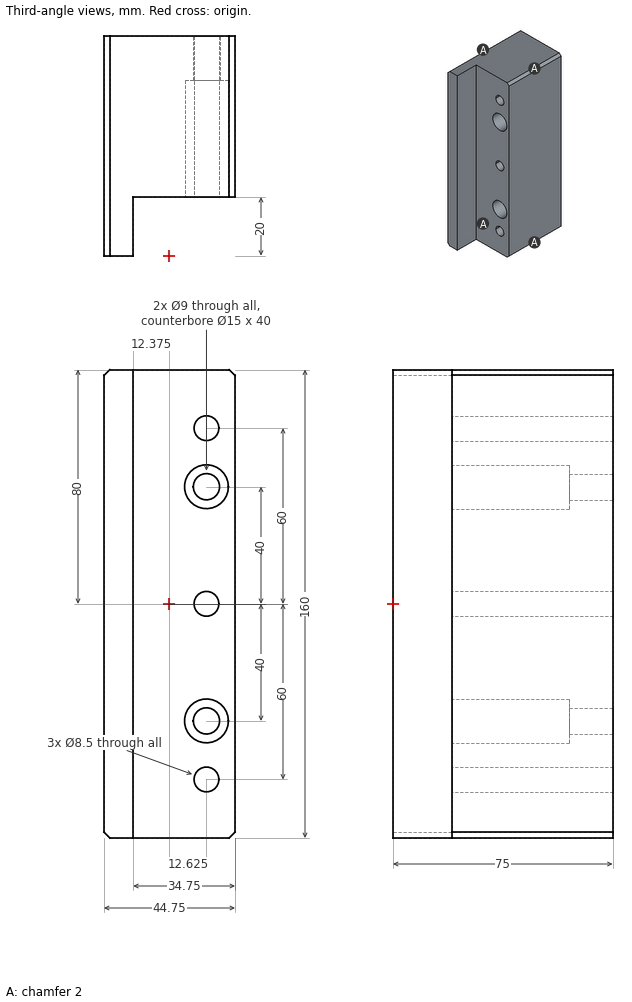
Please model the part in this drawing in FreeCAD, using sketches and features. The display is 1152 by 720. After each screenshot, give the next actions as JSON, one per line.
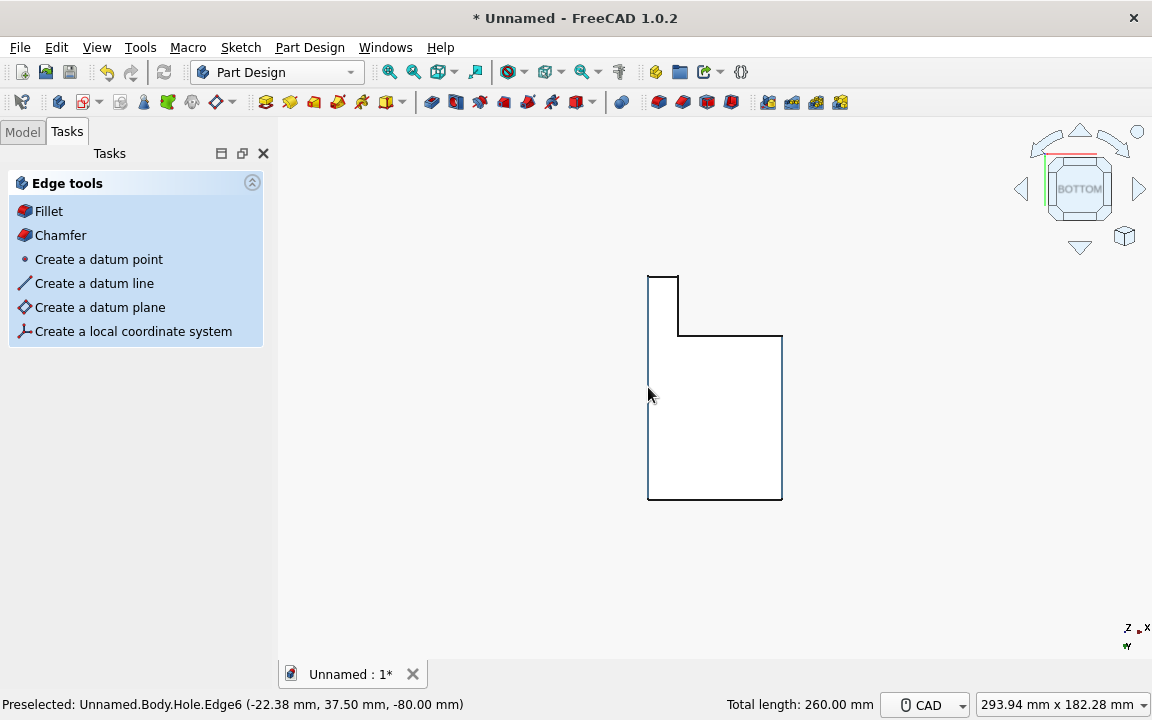
{"action": "left_click", "coordinate": [684, 102]}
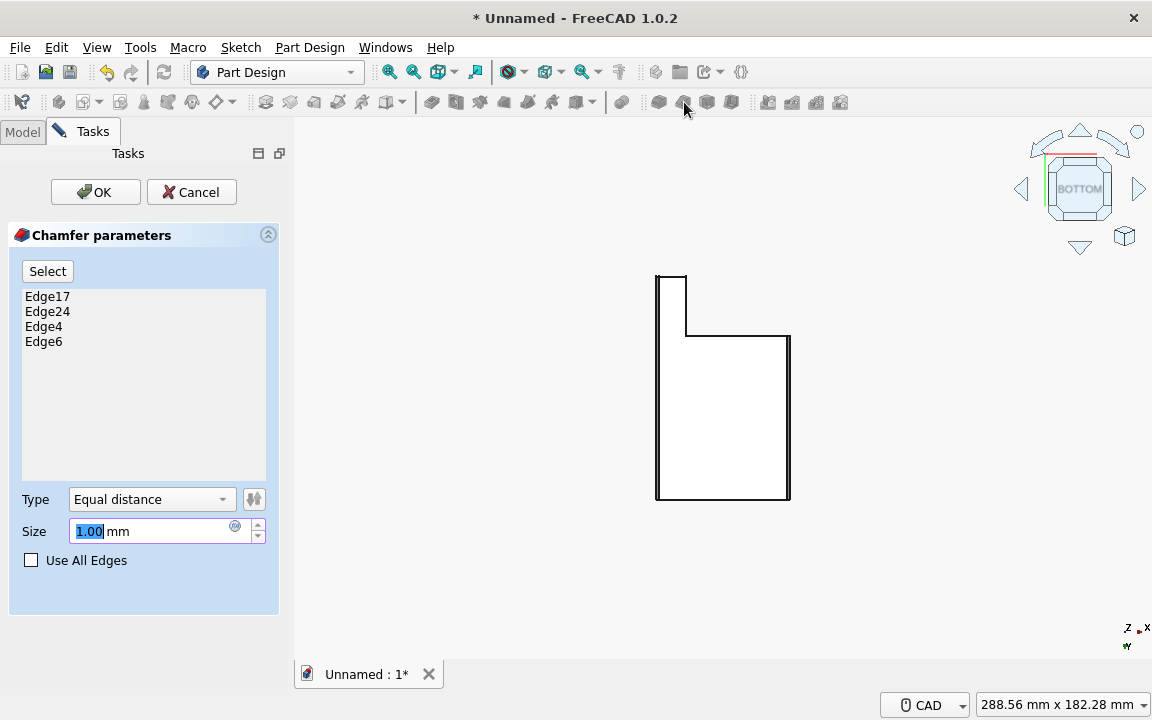
{"action": "type", "text": "2"}
{"action": "key", "text": "Tab"}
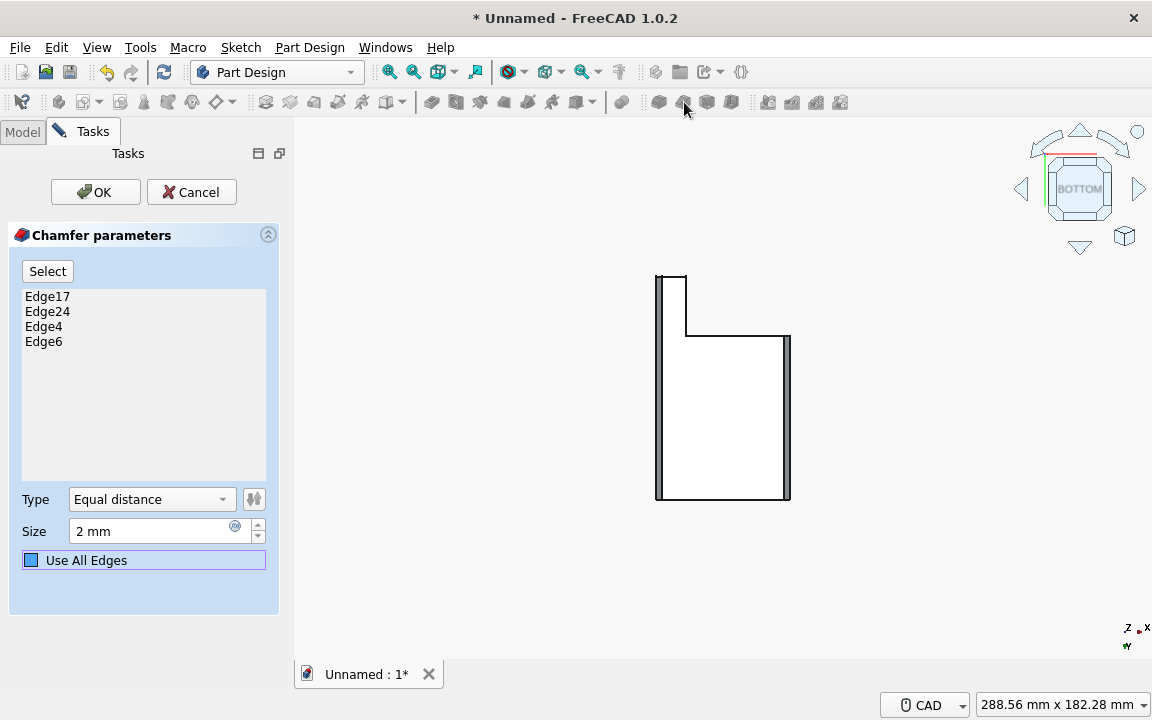
{"action": "left_click", "coordinate": [96, 192]}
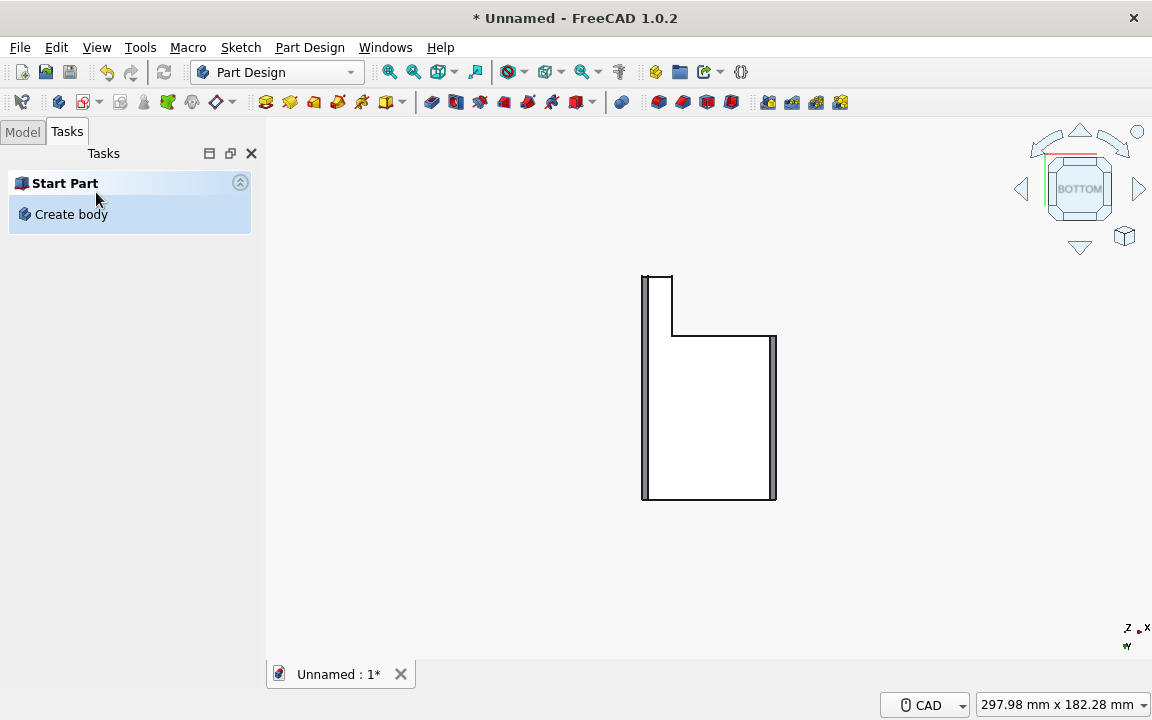
{"action": "left_click", "coordinate": [390, 72]}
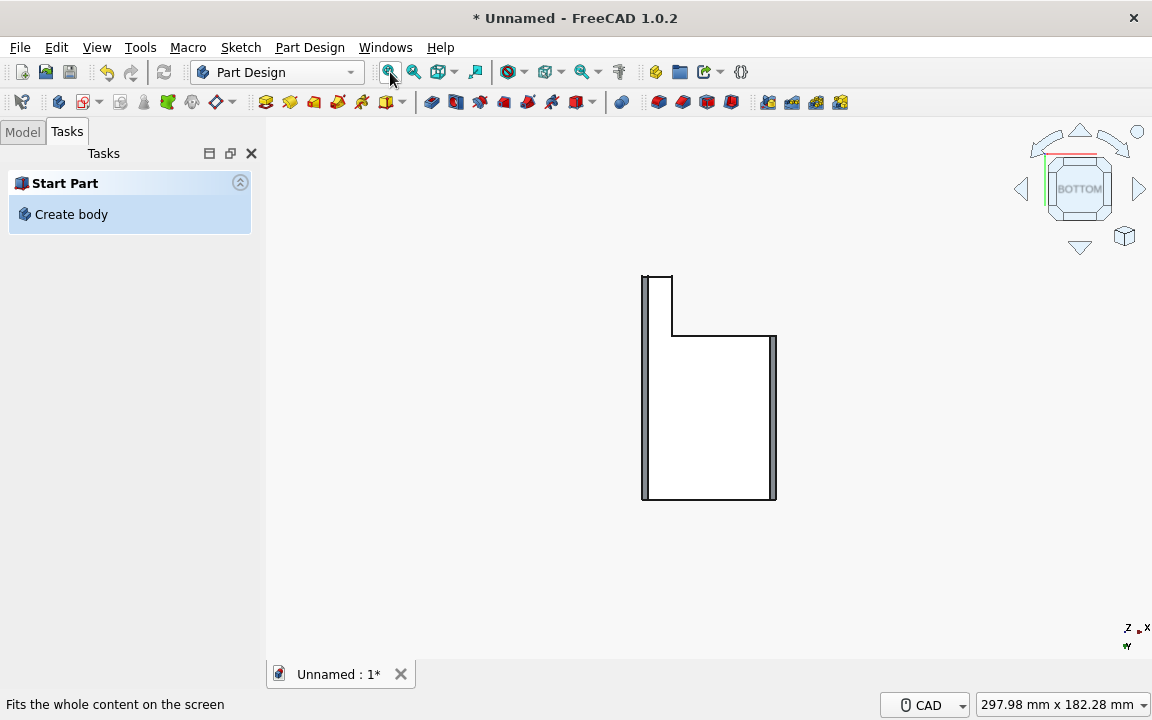
{"action": "key", "text": "0"}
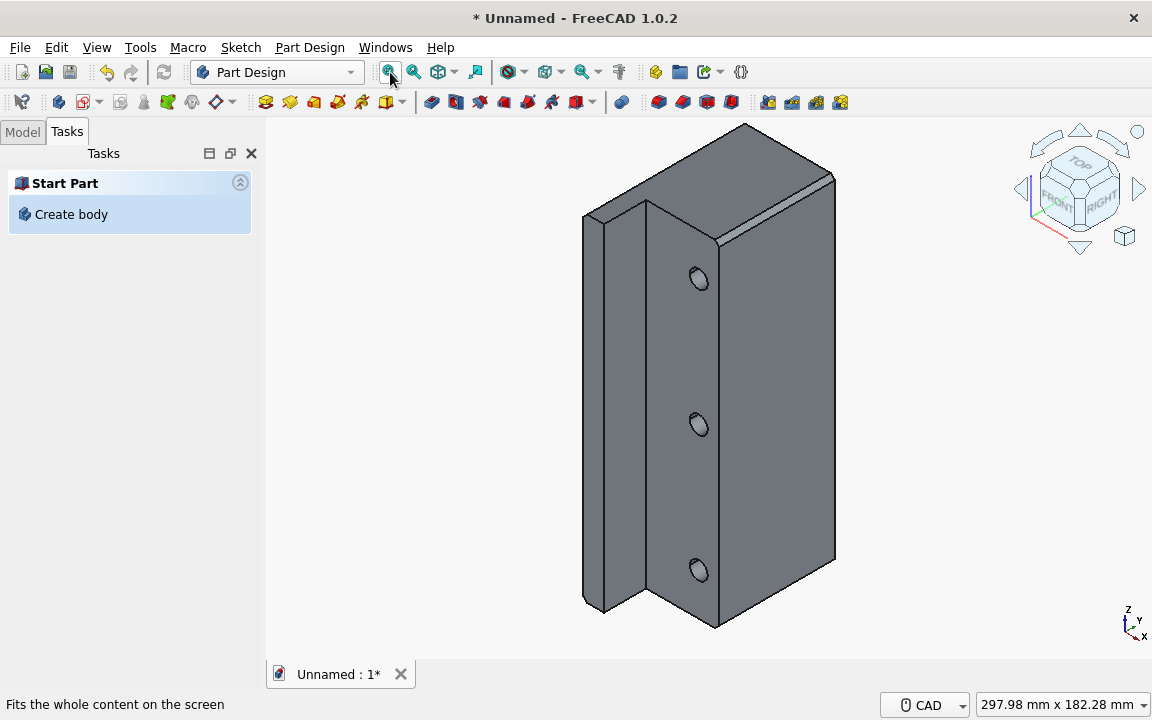
{"action": "left_click", "coordinate": [683, 359]}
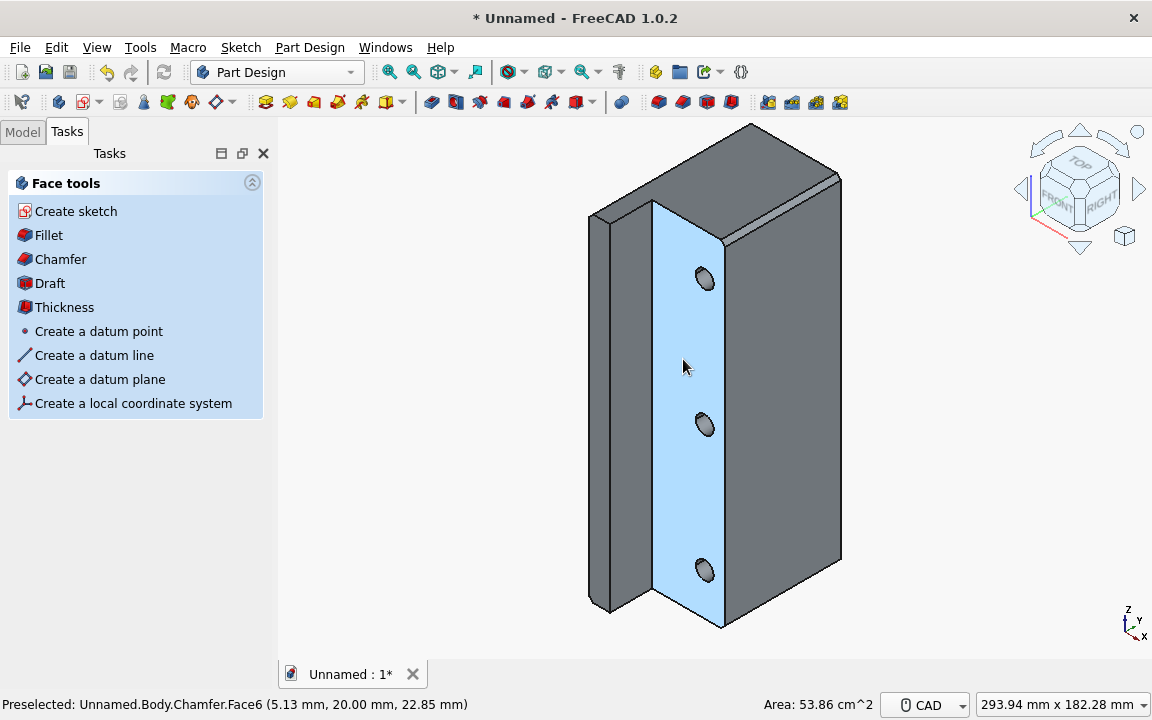
{"action": "left_click", "coordinate": [84, 102]}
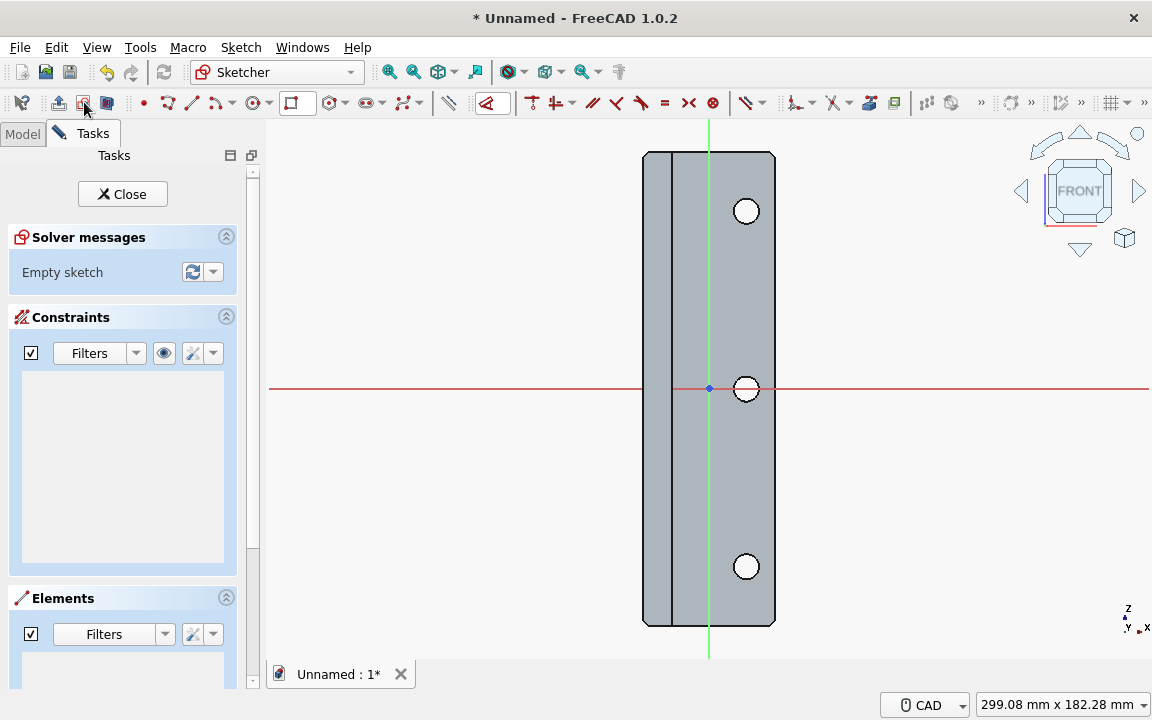
{"action": "left_click", "coordinate": [254, 104]}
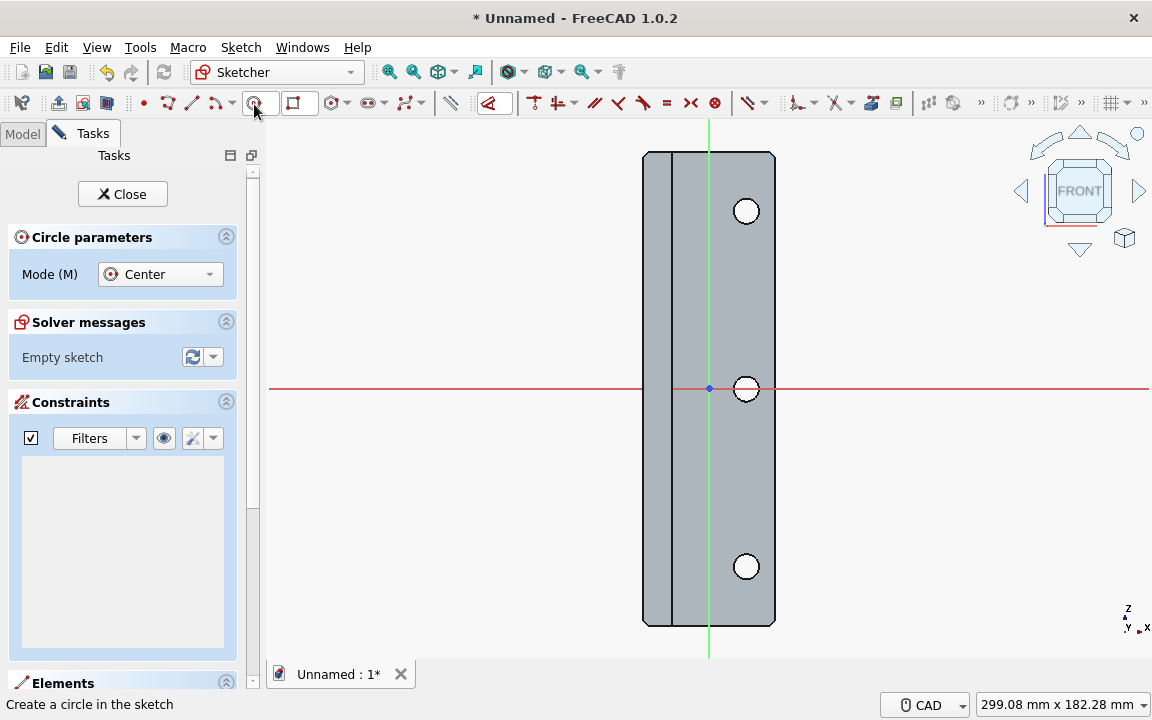
{"action": "scroll", "coordinate": [746, 271], "scroll_direction": "up", "scroll_amount": 3}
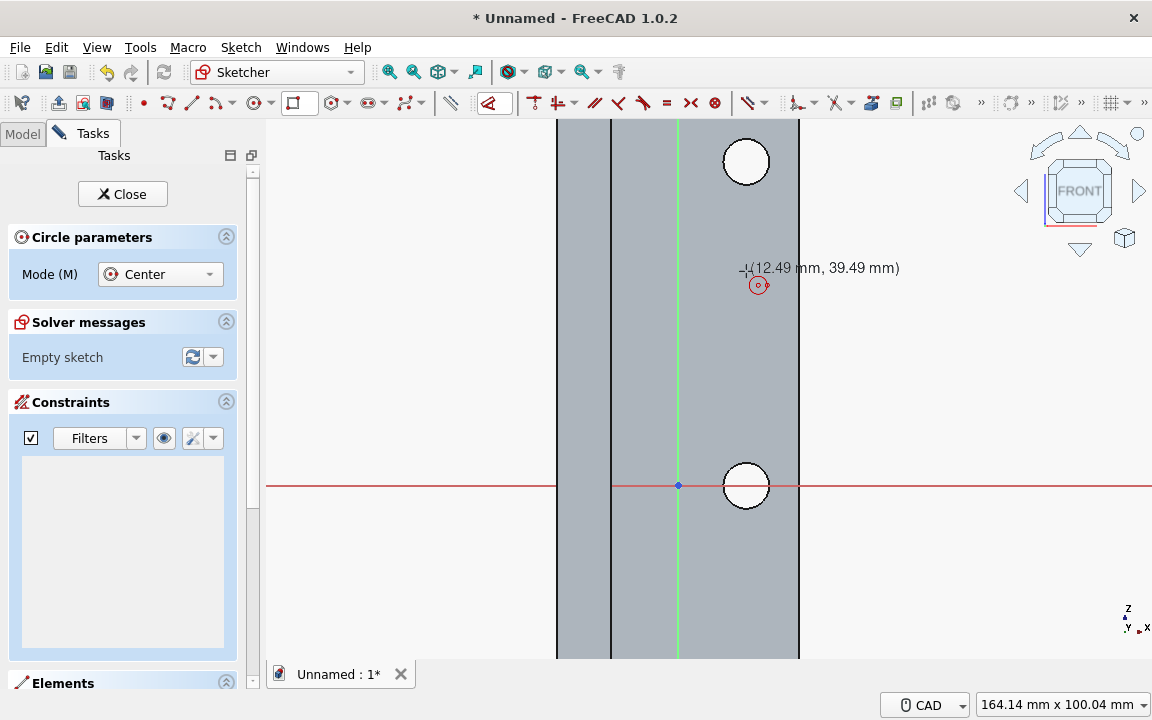
{"action": "left_click", "coordinate": [746, 270]}
{"action": "left_click", "coordinate": [763, 253]}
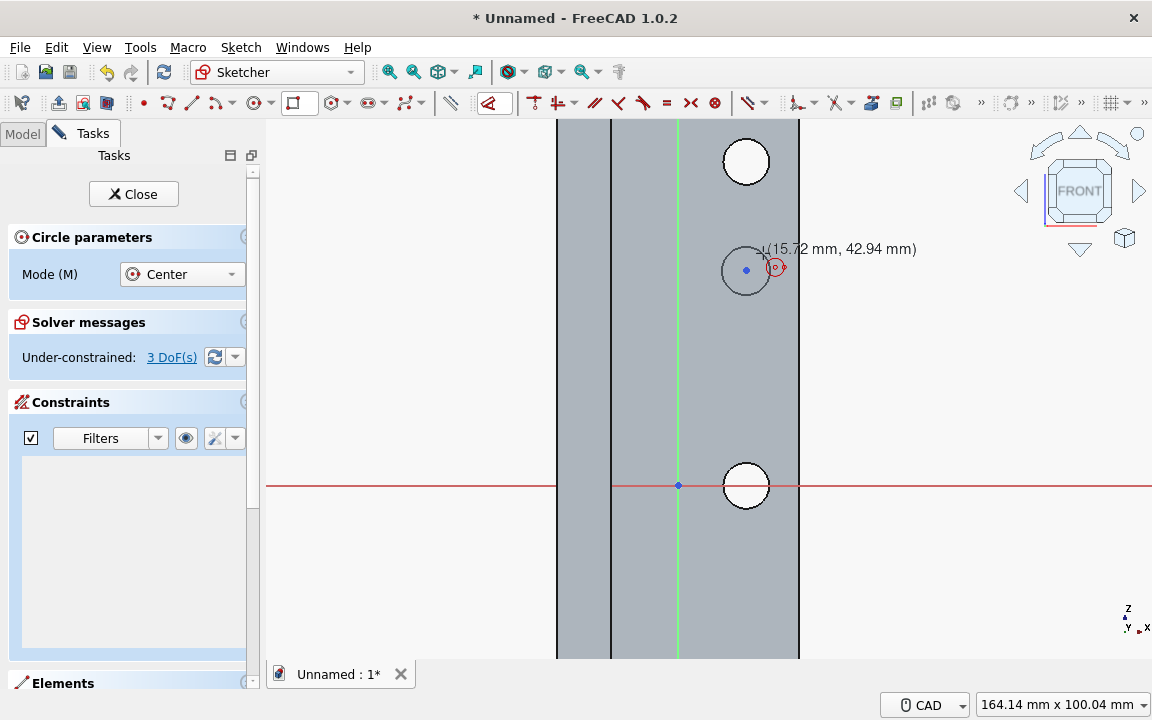
{"action": "scroll", "coordinate": [470, 192], "scroll_direction": "down", "scroll_amount": 2}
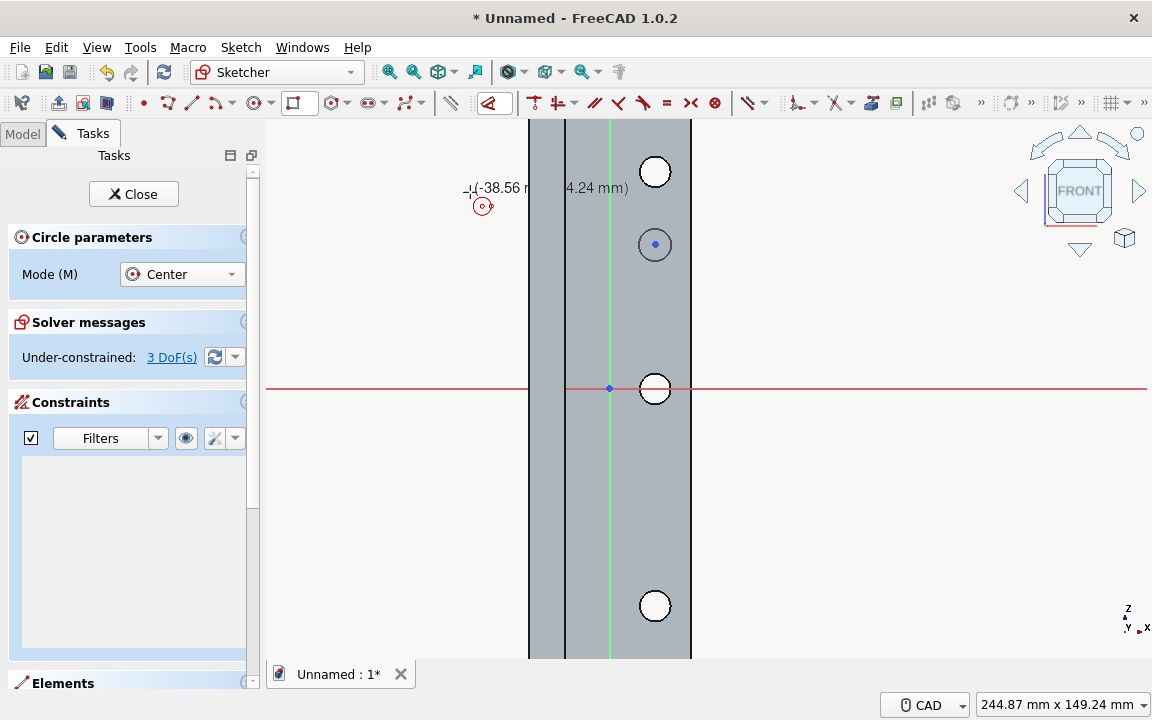
{"action": "scroll", "coordinate": [655, 534], "scroll_direction": "up", "scroll_amount": 2}